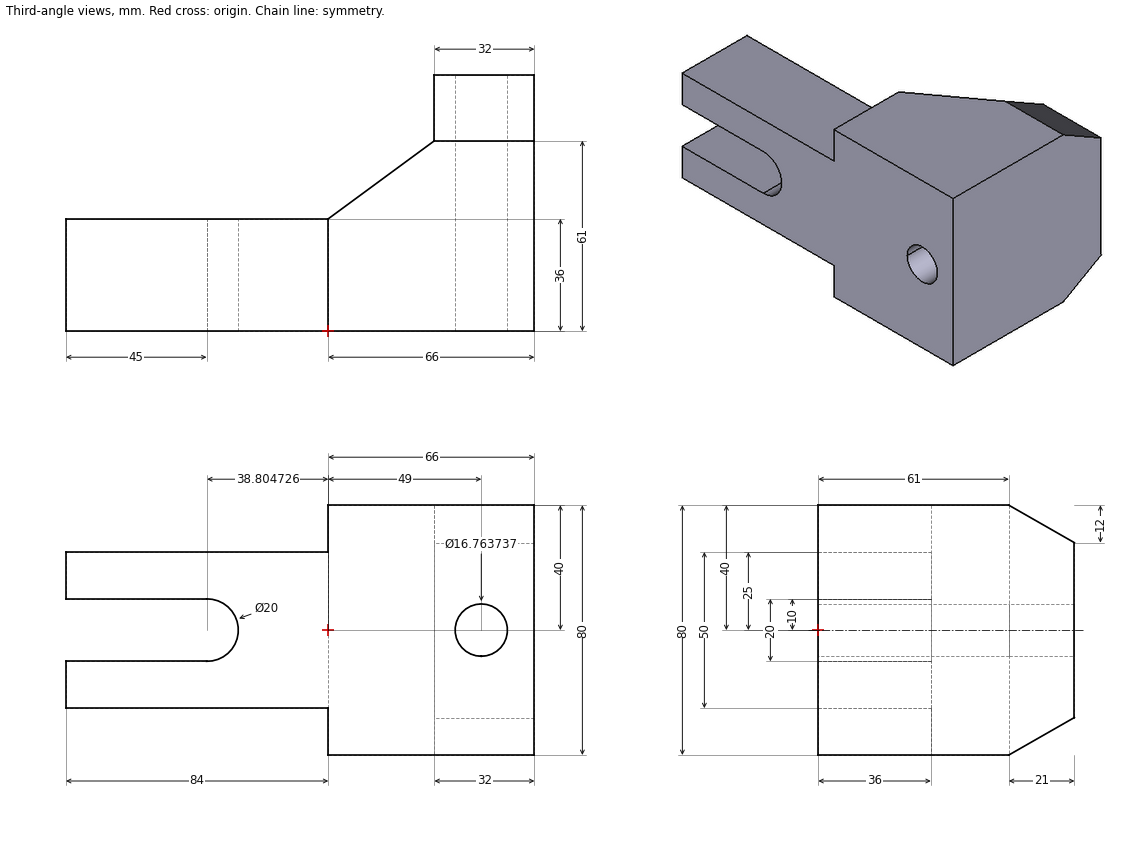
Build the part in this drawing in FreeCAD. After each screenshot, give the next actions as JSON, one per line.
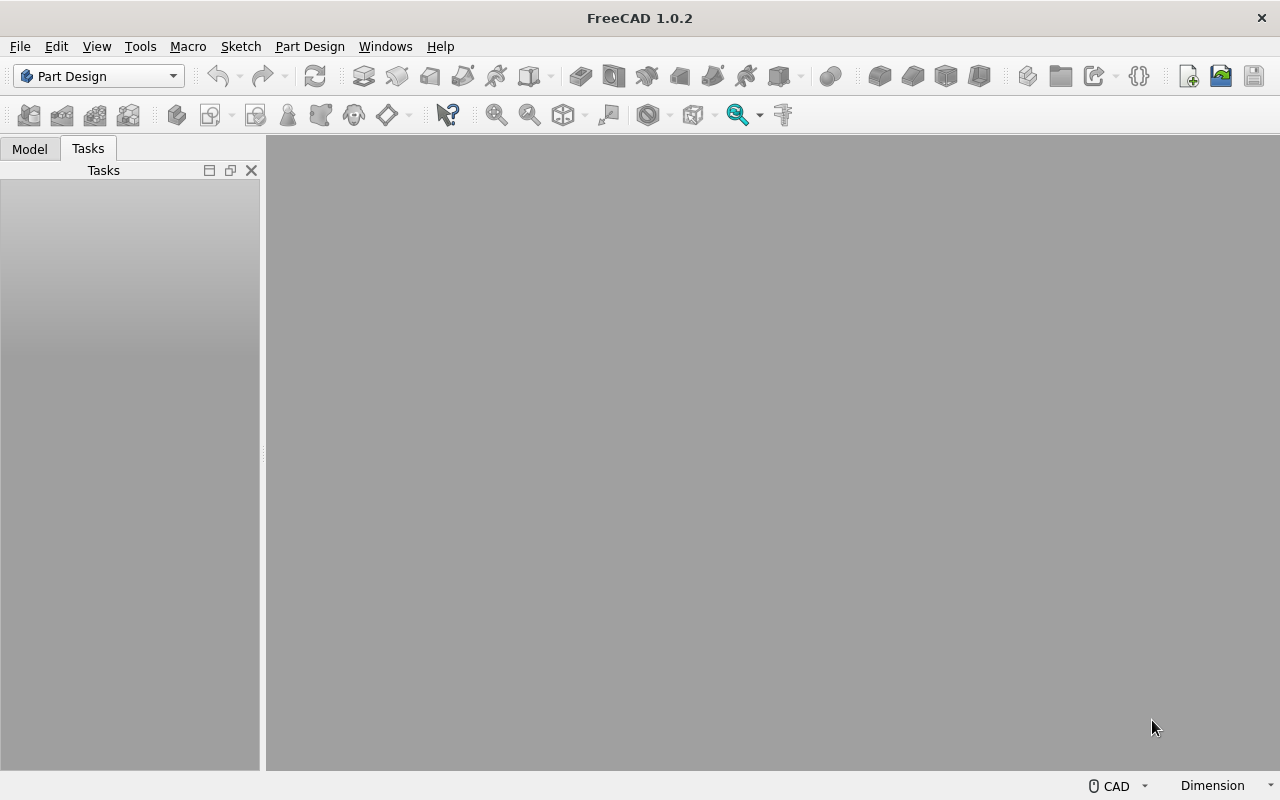
{"action": "key", "text": "ctrl+n"}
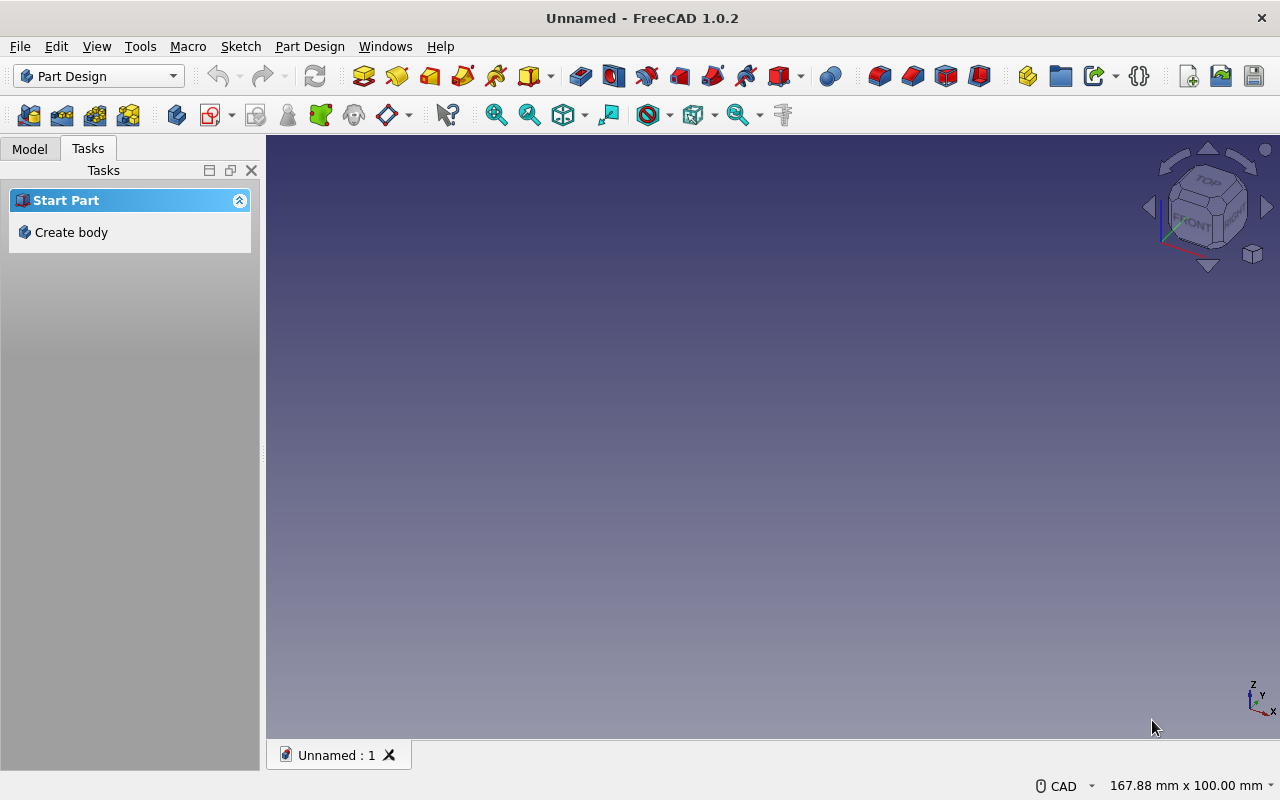
{"action": "left_click", "coordinate": [210, 116]}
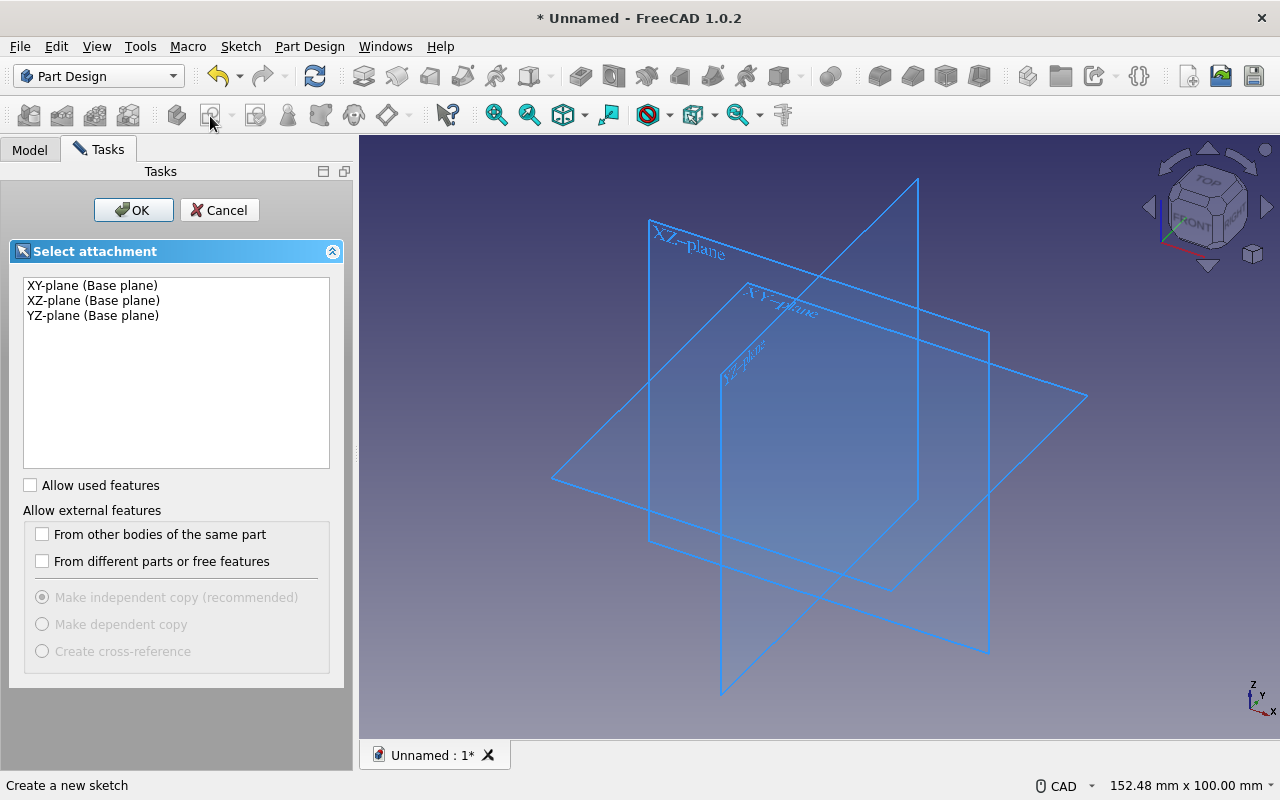
{"action": "left_click", "coordinate": [84, 286]}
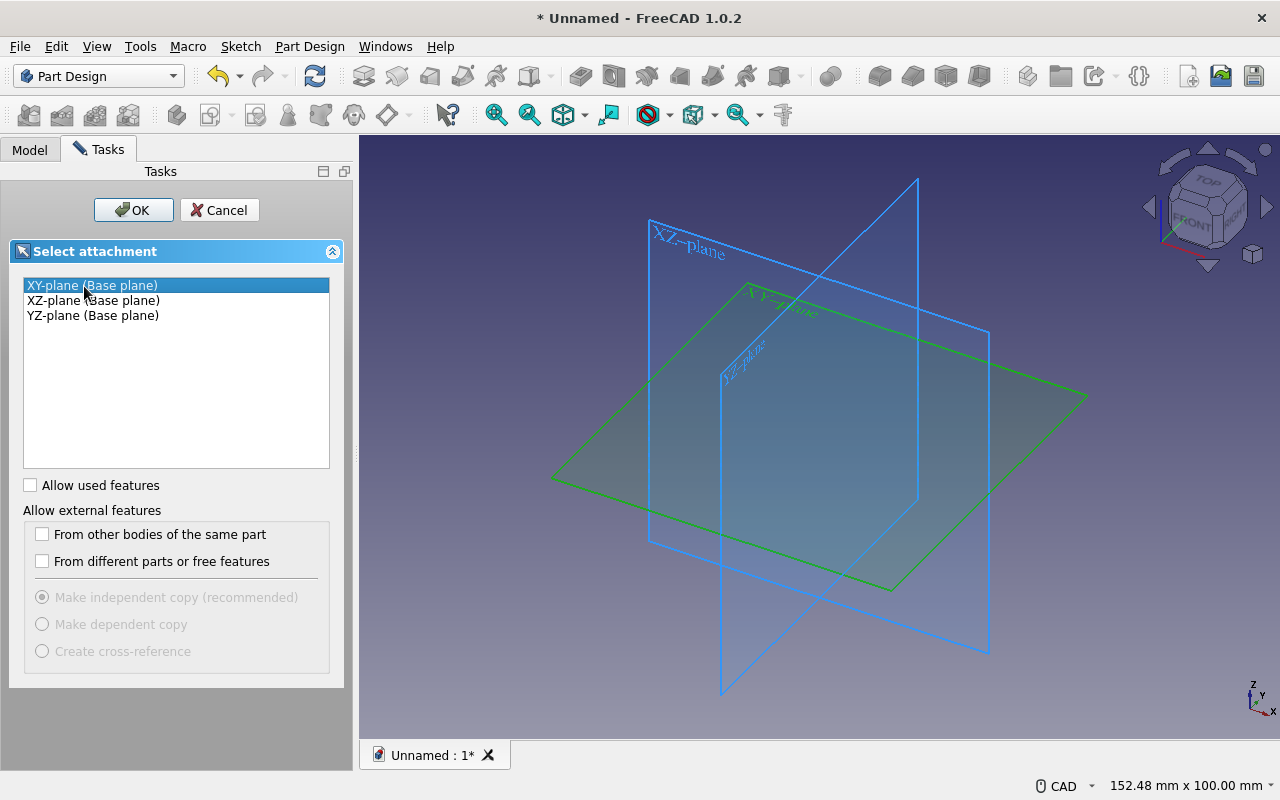
{"action": "left_click", "coordinate": [134, 210]}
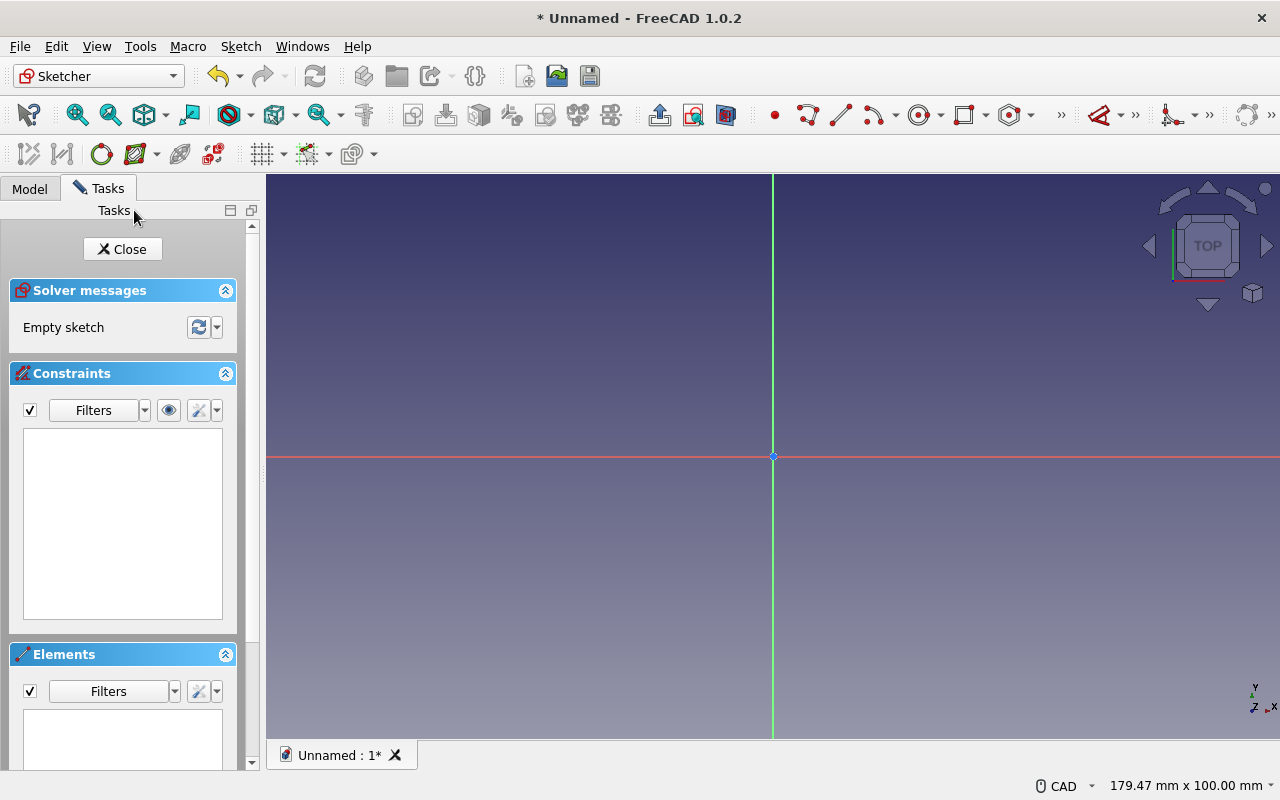
{"action": "scroll", "coordinate": [294, 711], "scroll_direction": "down", "scroll_amount": 2}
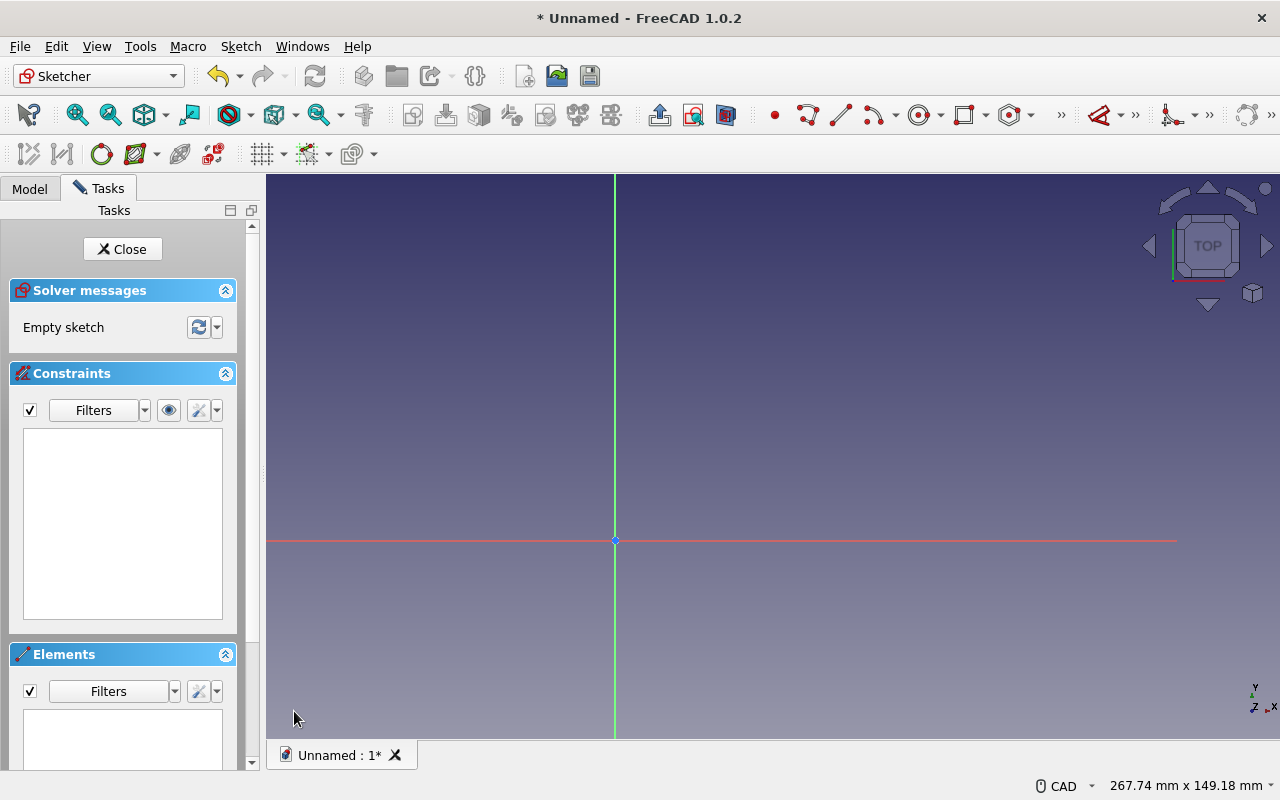
{"action": "scroll", "coordinate": [812, 362], "scroll_direction": "up", "scroll_amount": 2}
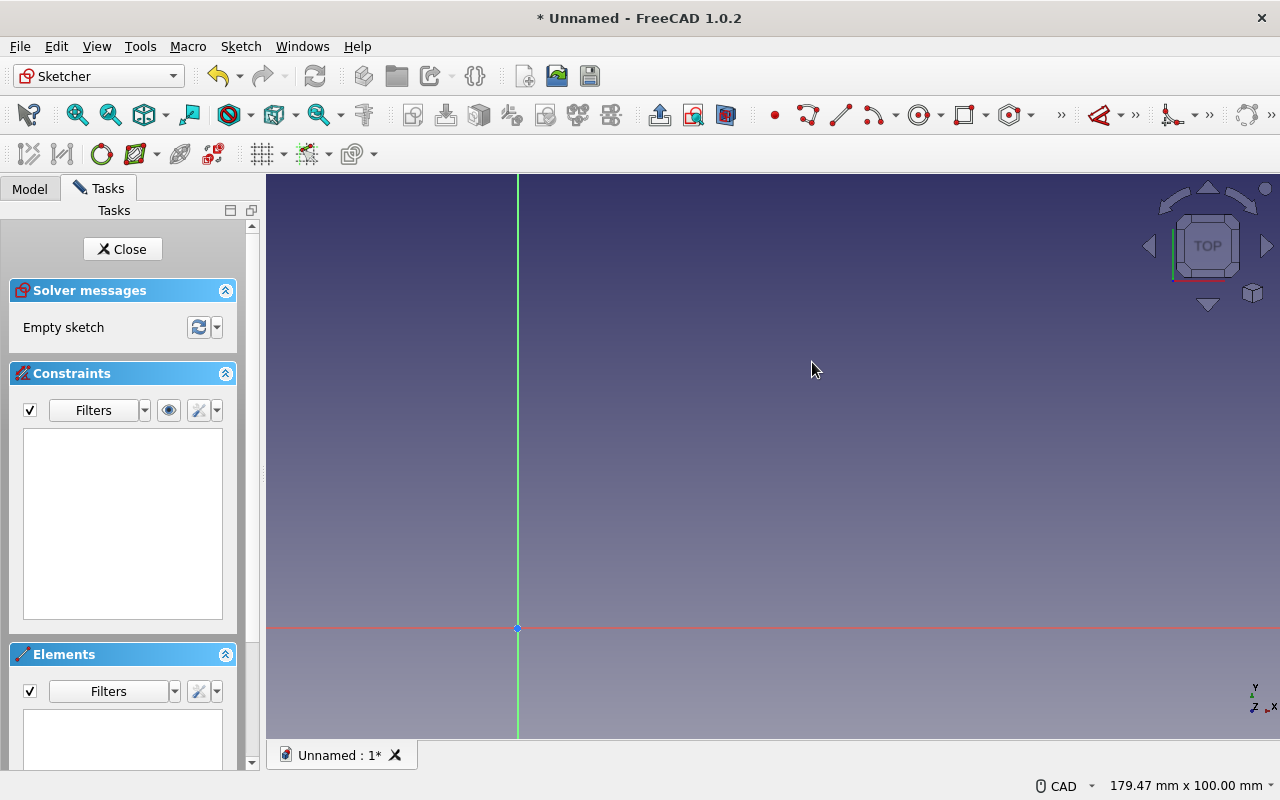
{"action": "key", "text": "g m"}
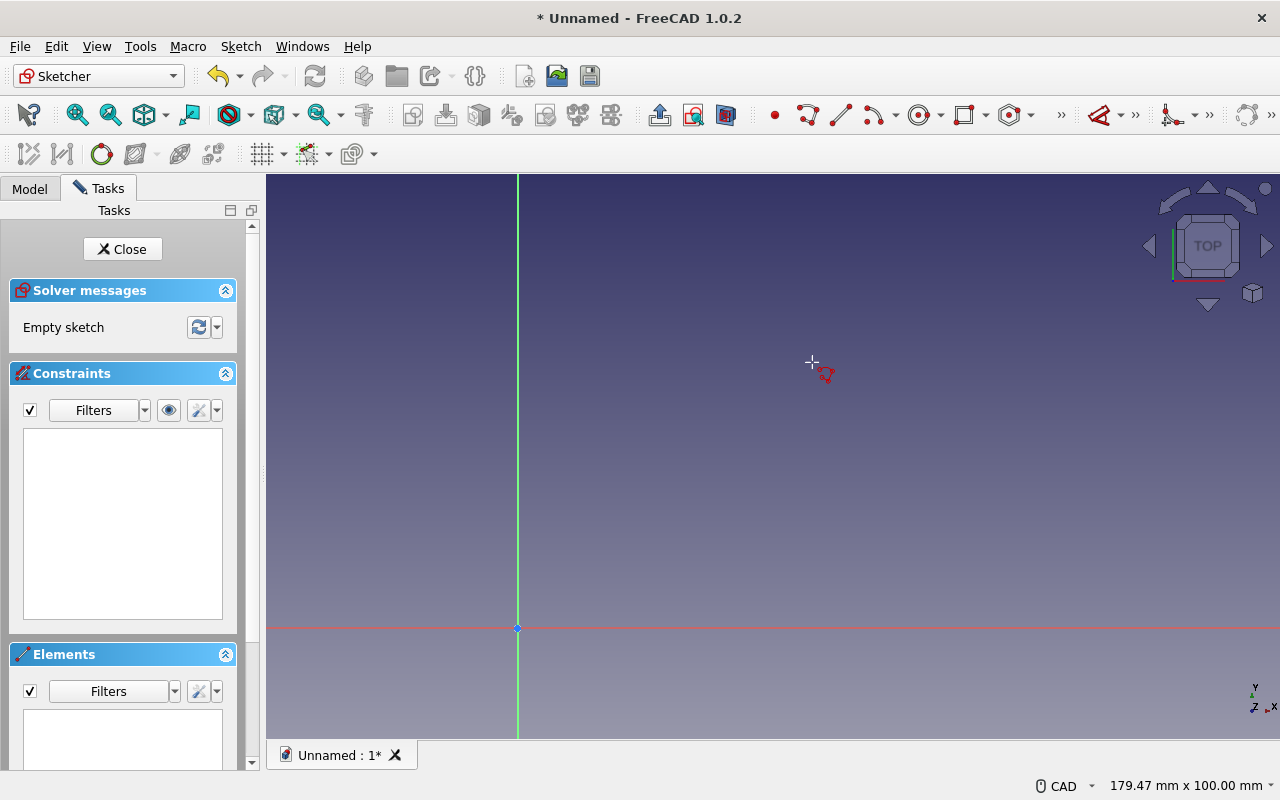
{"action": "left_click", "coordinate": [518, 628]}
{"action": "left_click", "coordinate": [891, 619]}
{"action": "left_click", "coordinate": [891, 284]}
{"action": "left_click", "coordinate": [710, 284]}
{"action": "left_click", "coordinate": [527, 425]}
{"action": "left_click", "coordinate": [518, 628]}
{"action": "key", "text": "Escape"}
{"action": "key", "text": "Escape"}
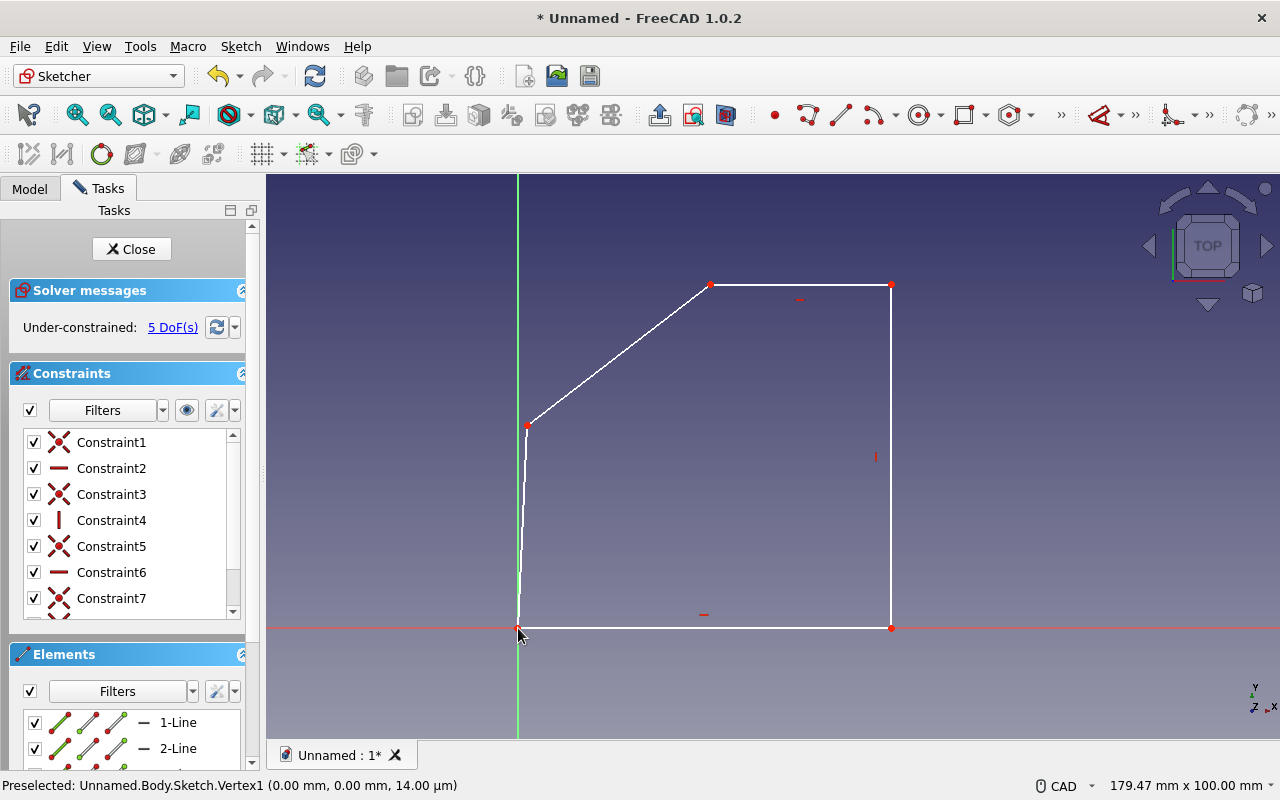
{"action": "left_click", "coordinate": [521, 568]}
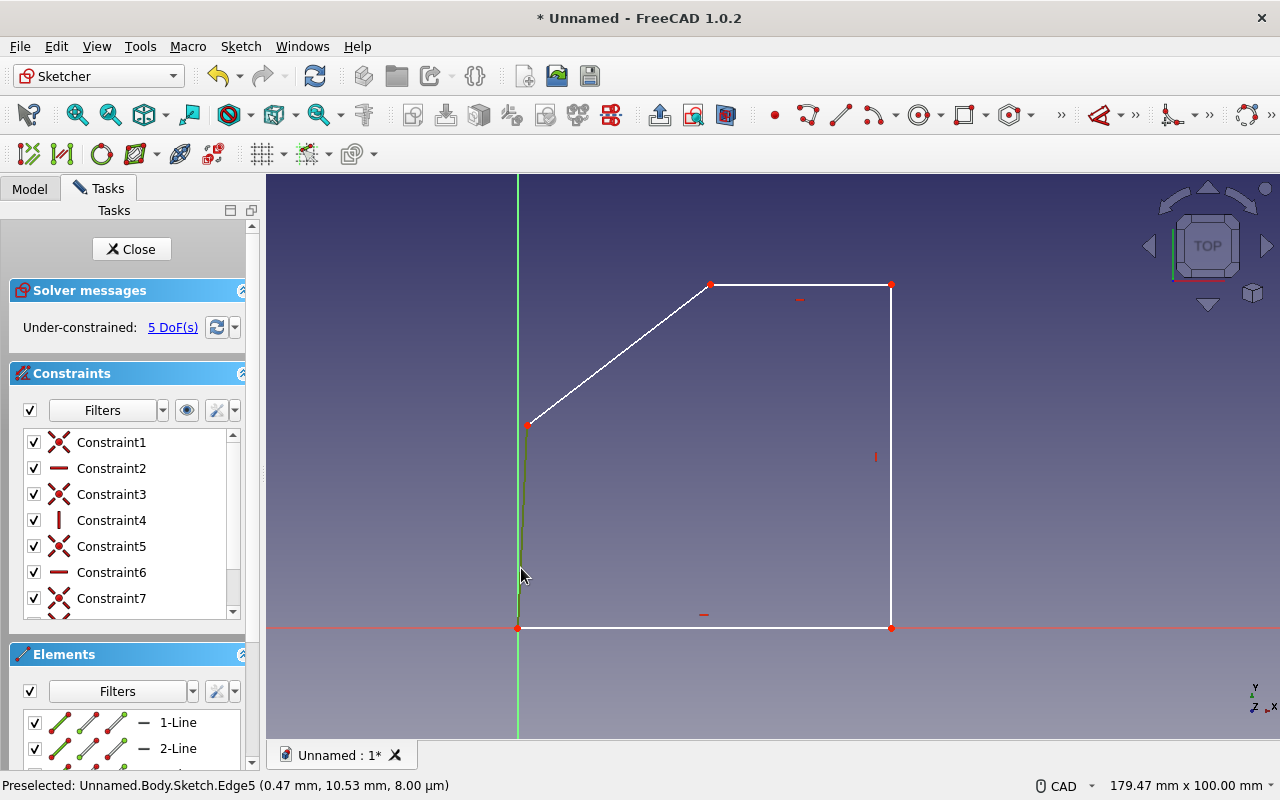
{"action": "key", "text": "v"}